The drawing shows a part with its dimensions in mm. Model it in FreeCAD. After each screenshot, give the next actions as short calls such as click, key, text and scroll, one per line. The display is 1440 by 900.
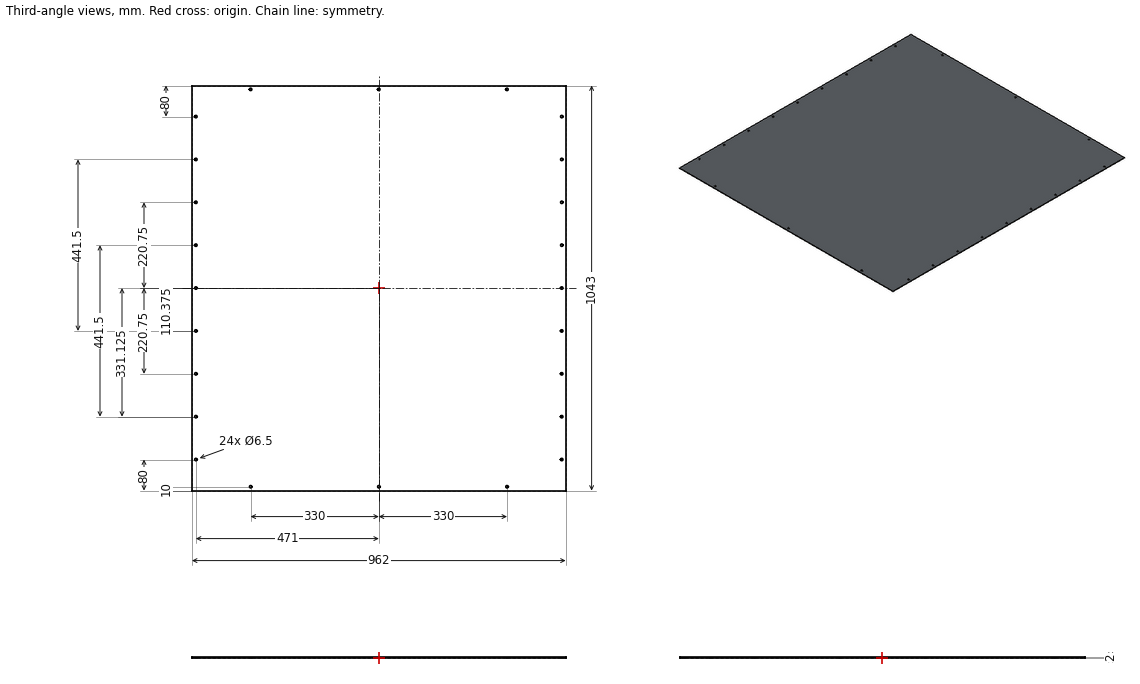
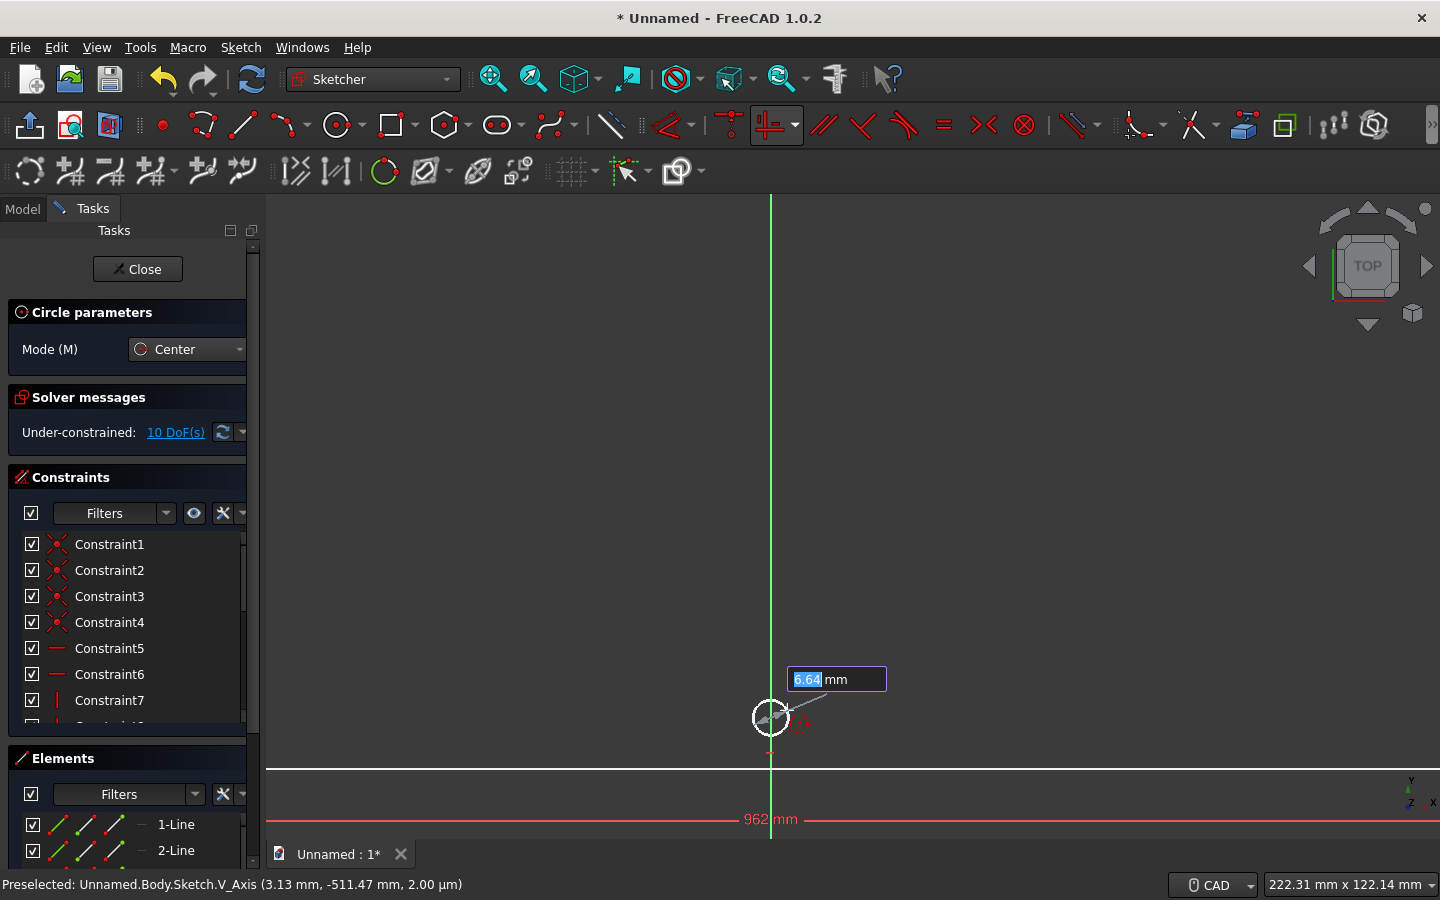
text(6.5)
key(Return)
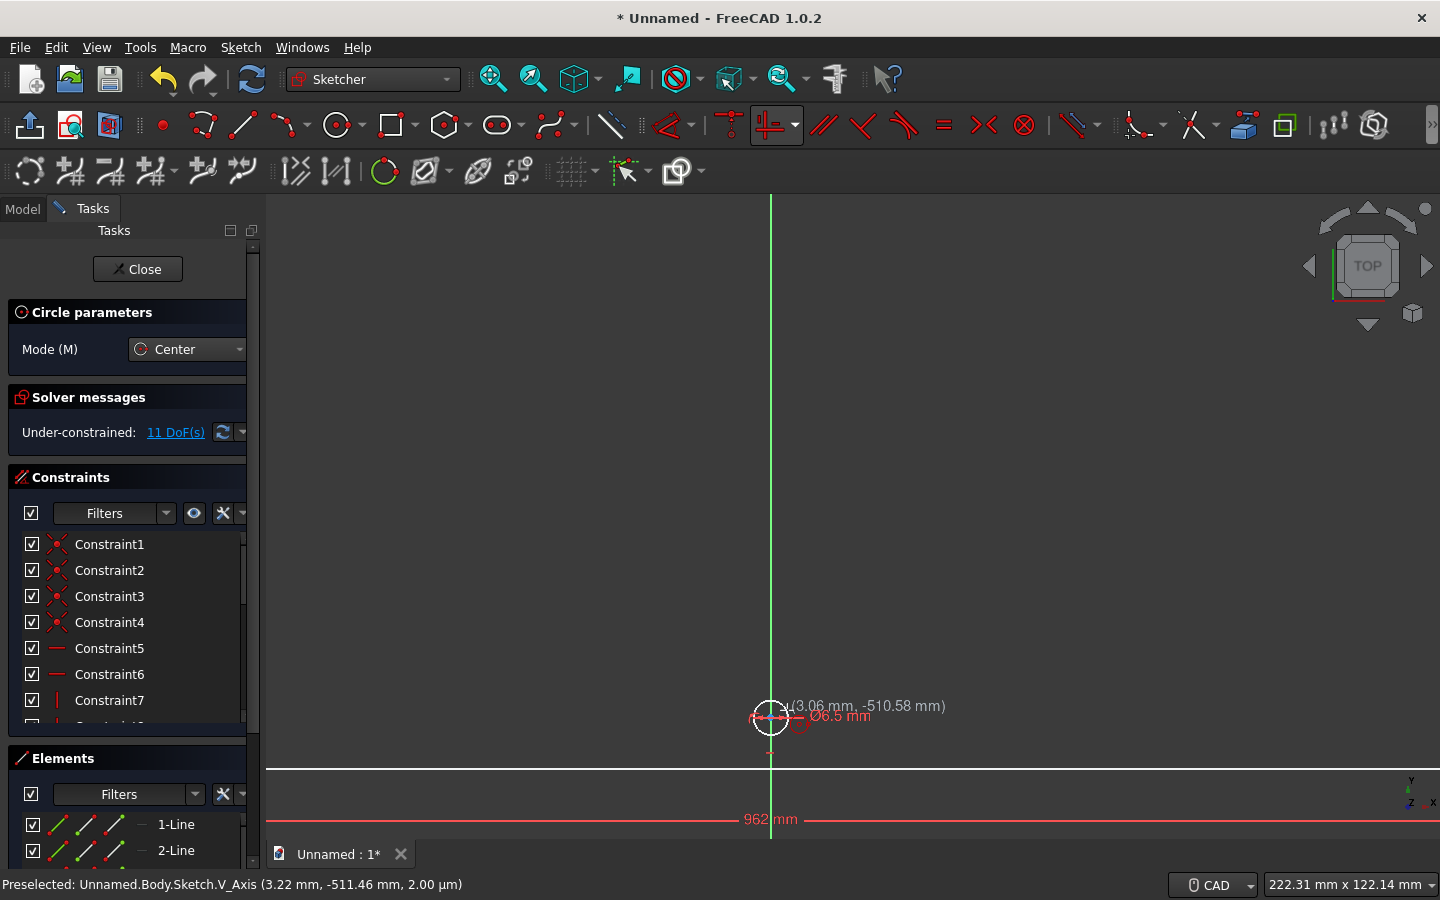
scroll(786, 717, down, 13)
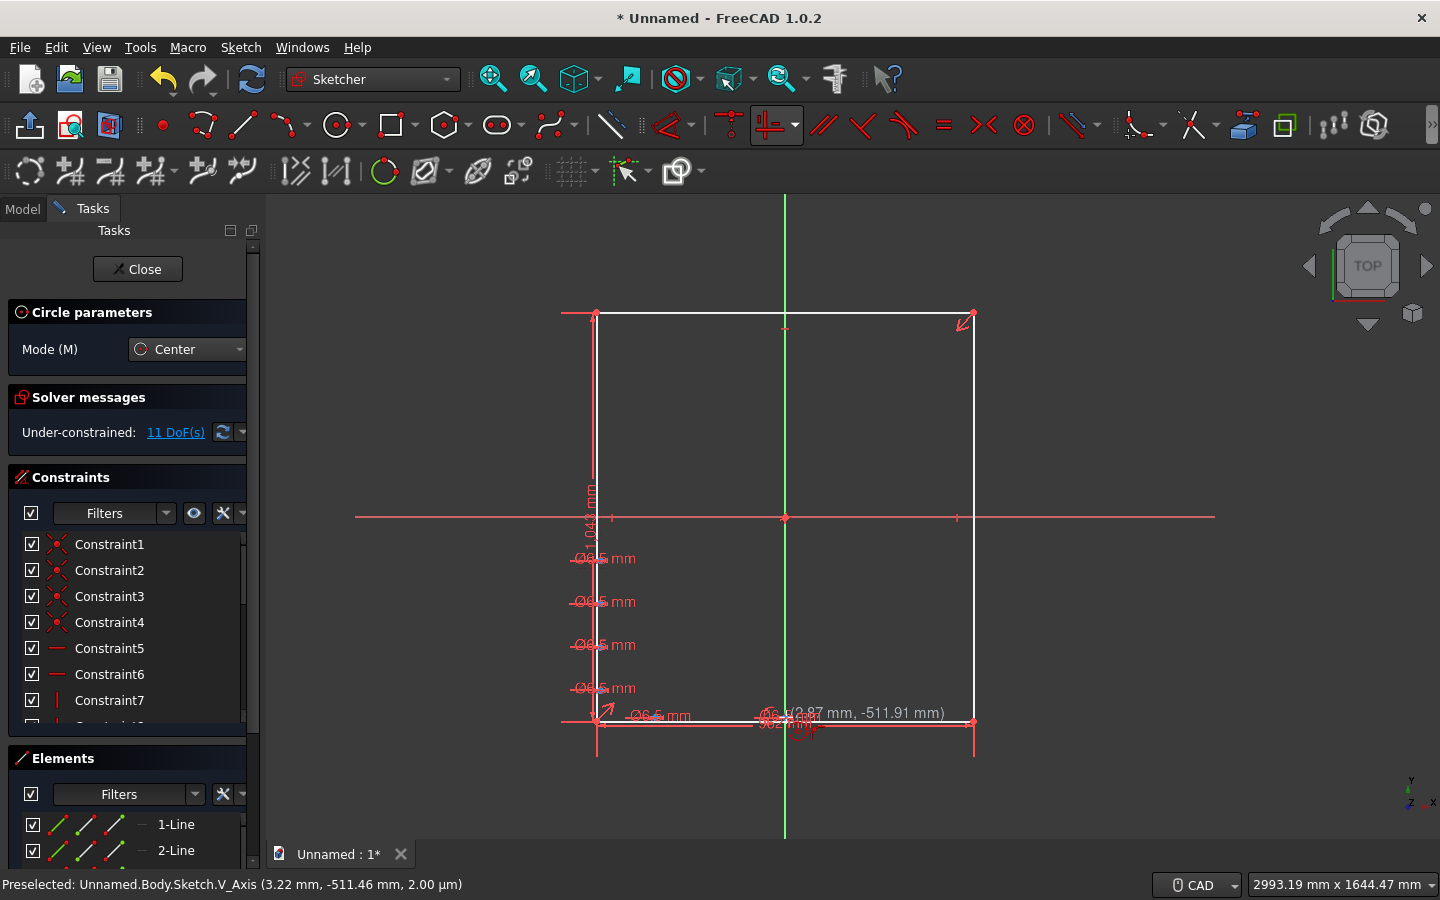
scroll(915, 718, up, 15)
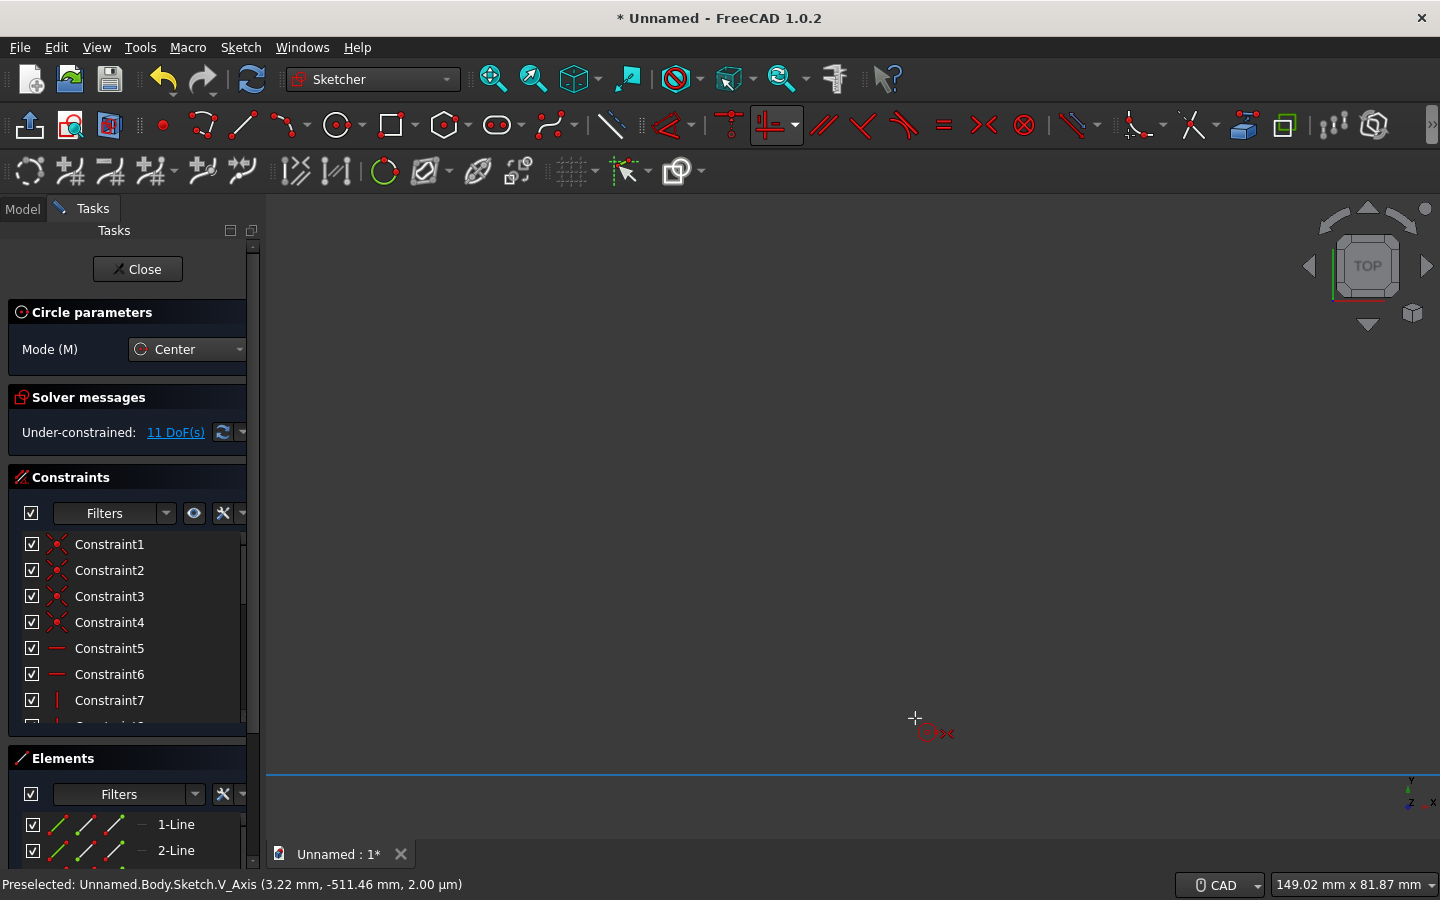
scroll(915, 718, down, 15)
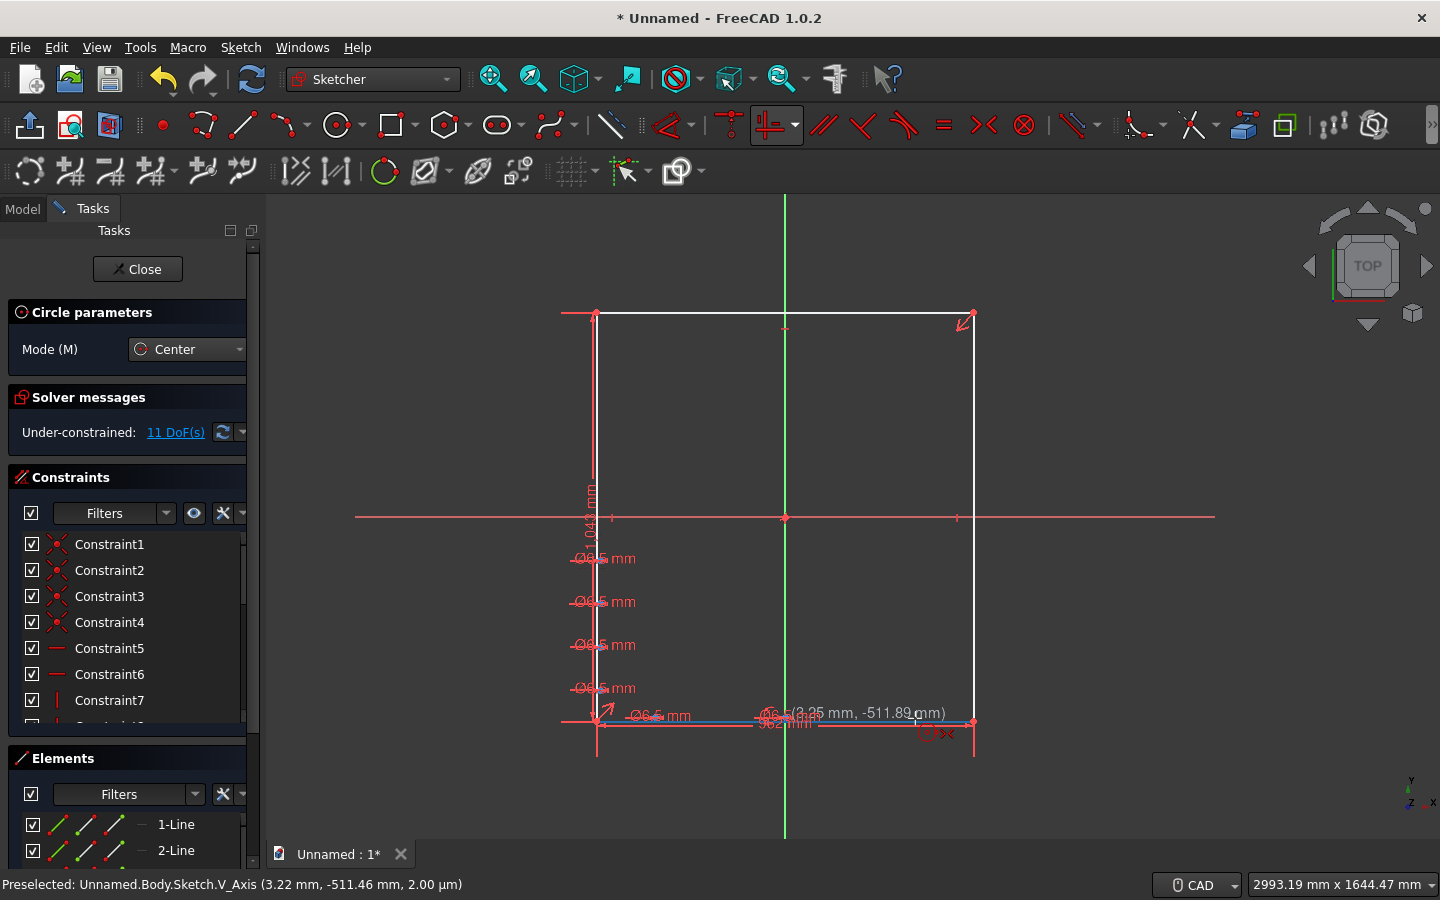
scroll(915, 718, up, 7)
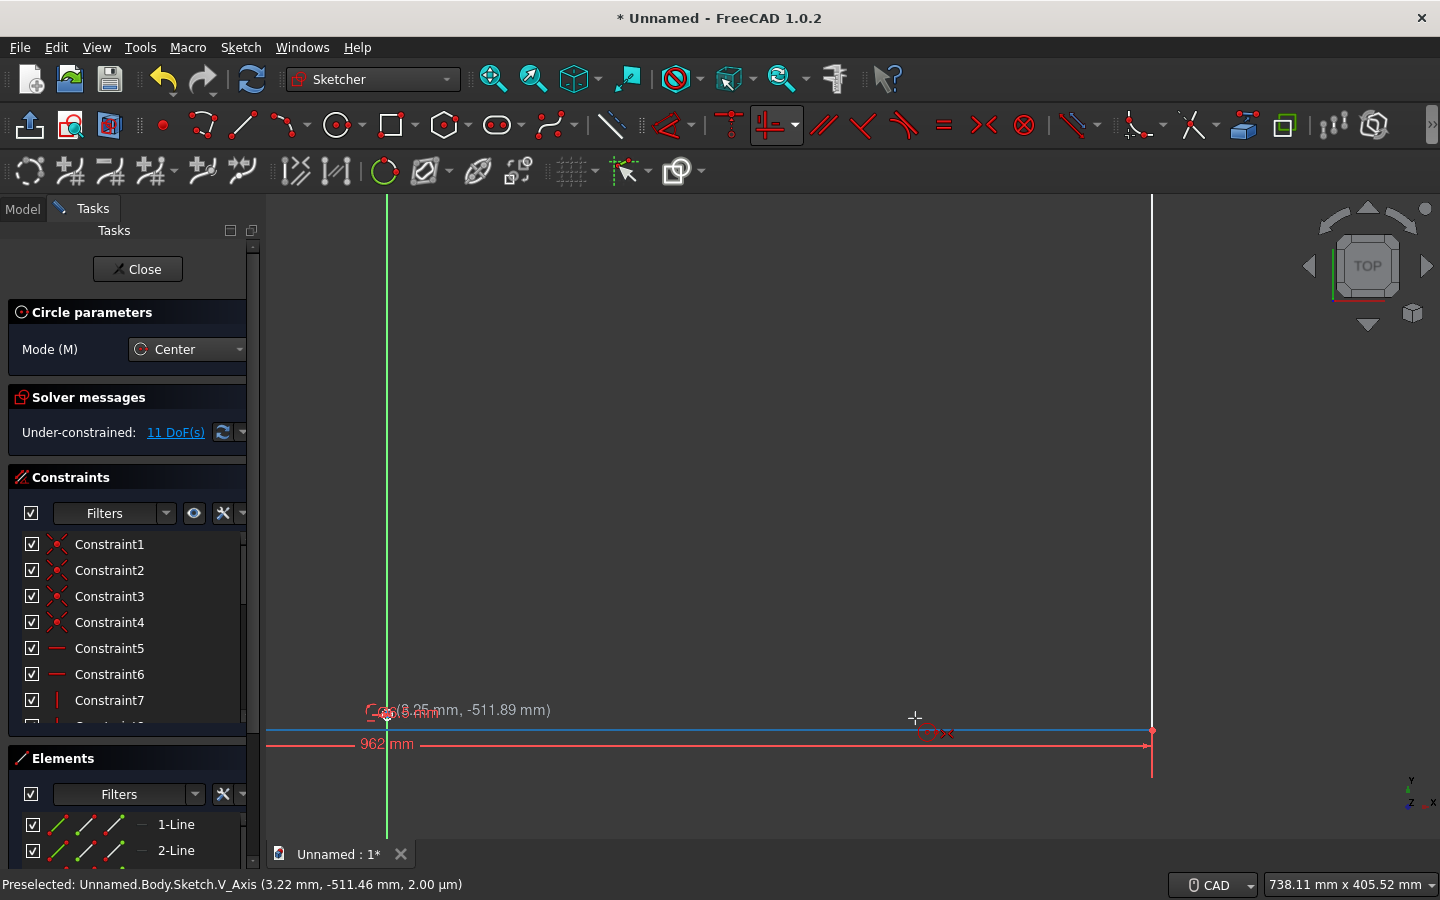
click(912, 714)
move(916, 711)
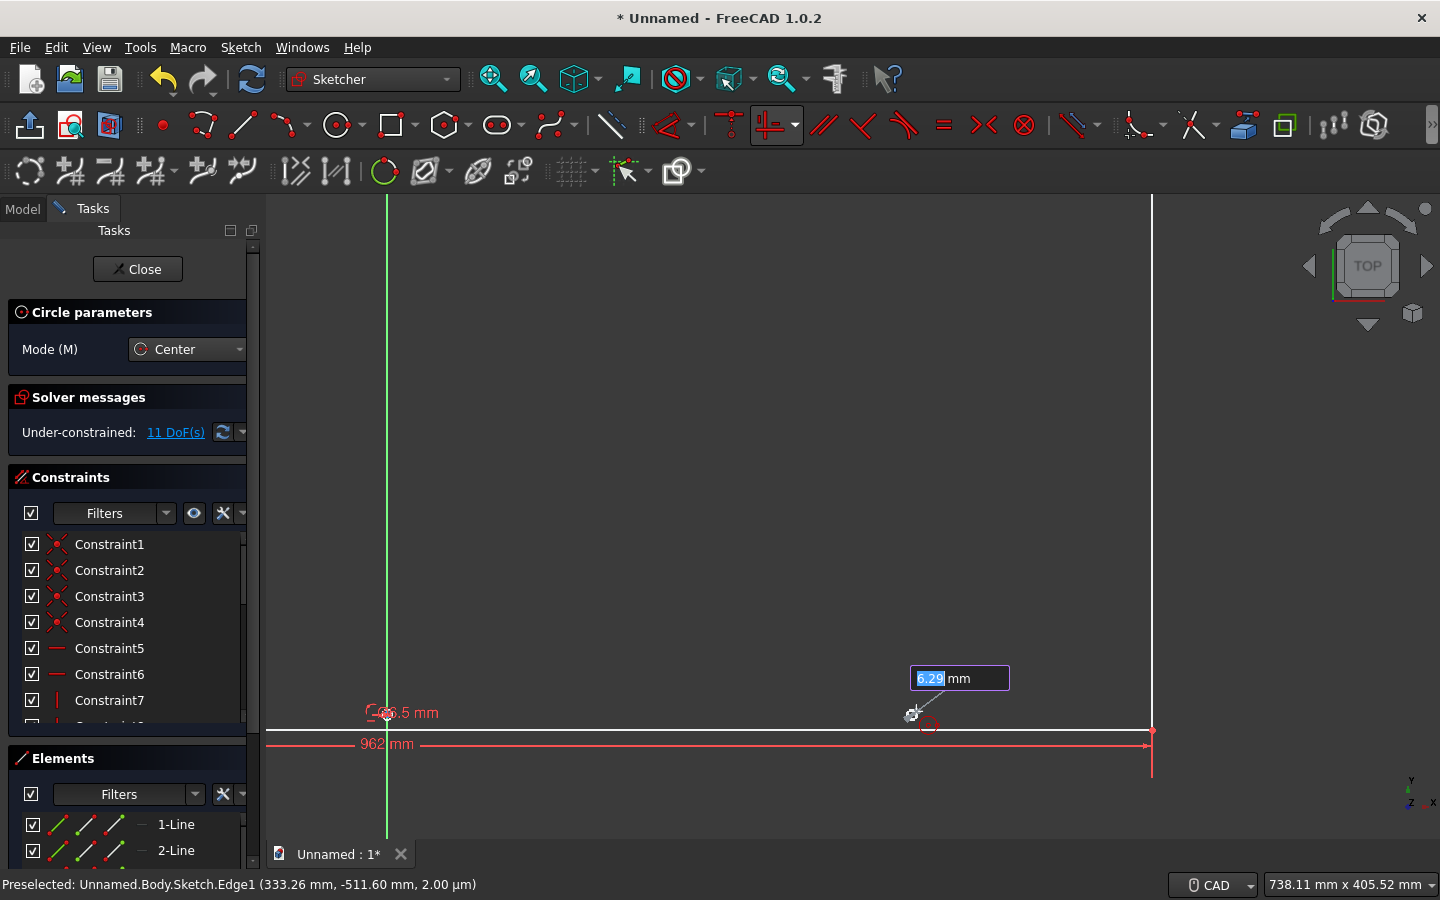
text(6.5)
key(Return)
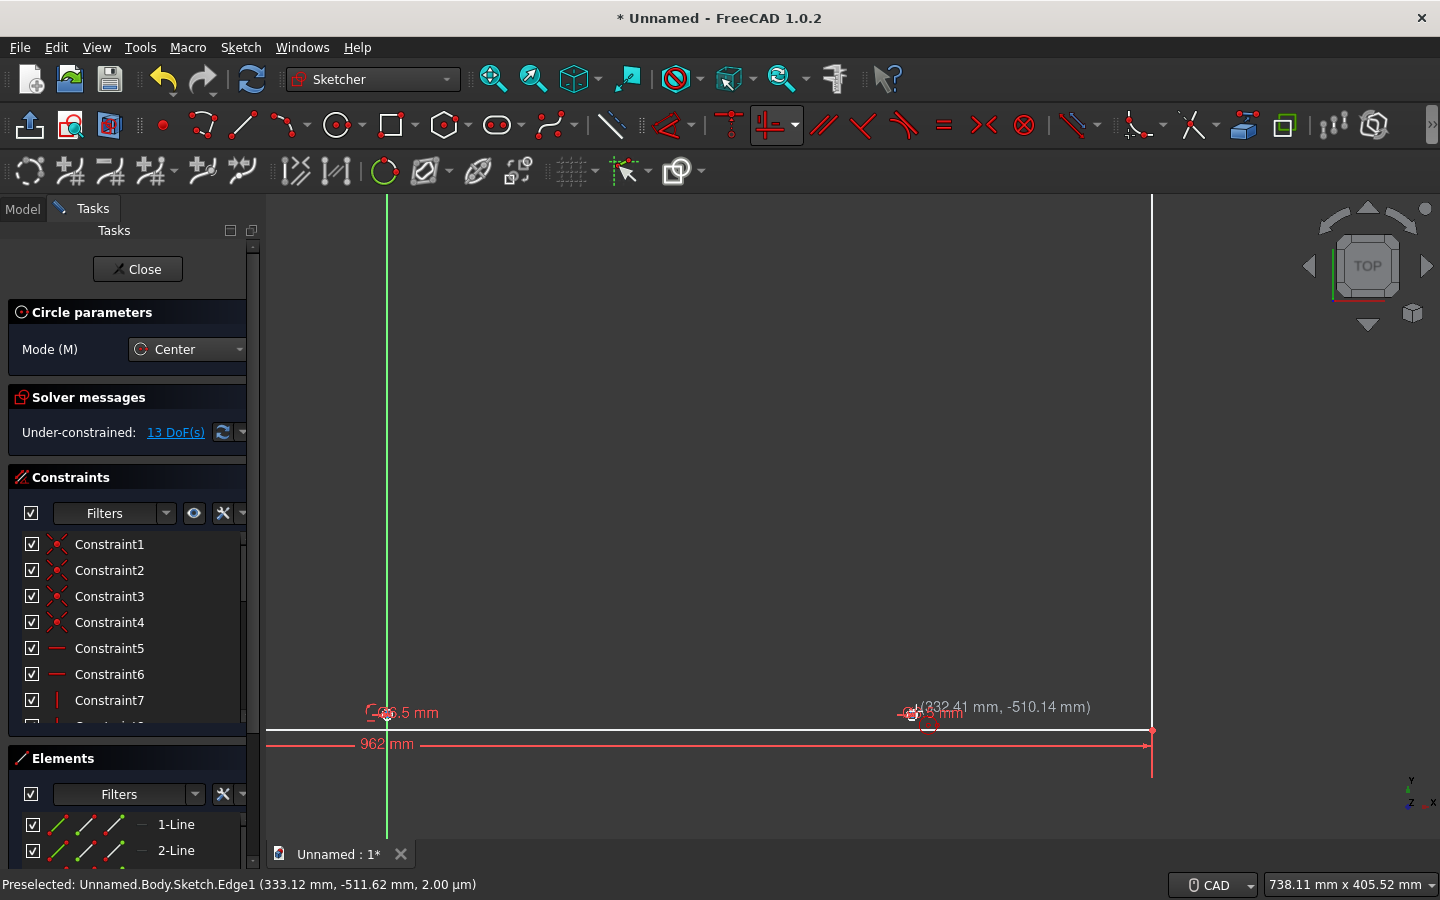
scroll(1136, 603, up, 8)